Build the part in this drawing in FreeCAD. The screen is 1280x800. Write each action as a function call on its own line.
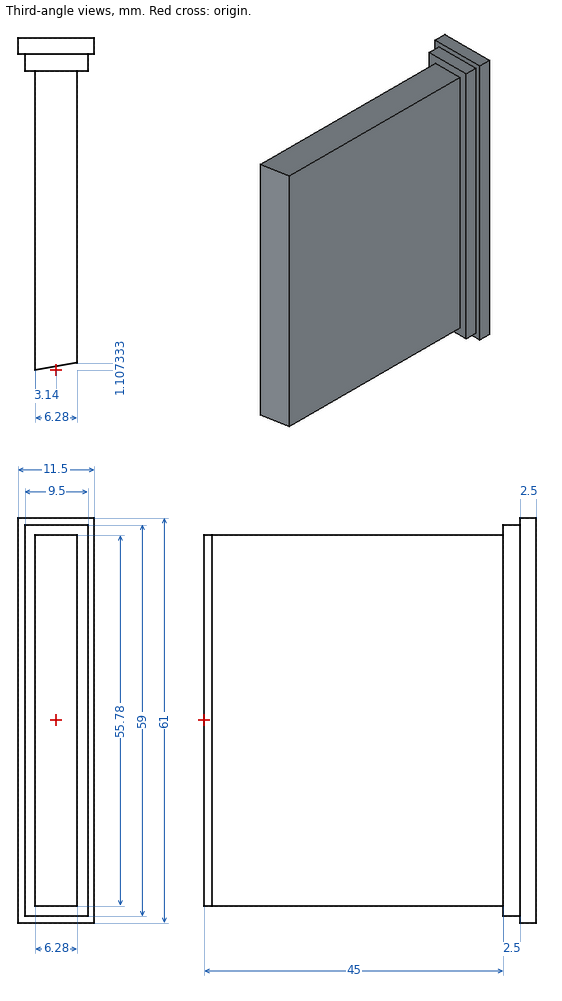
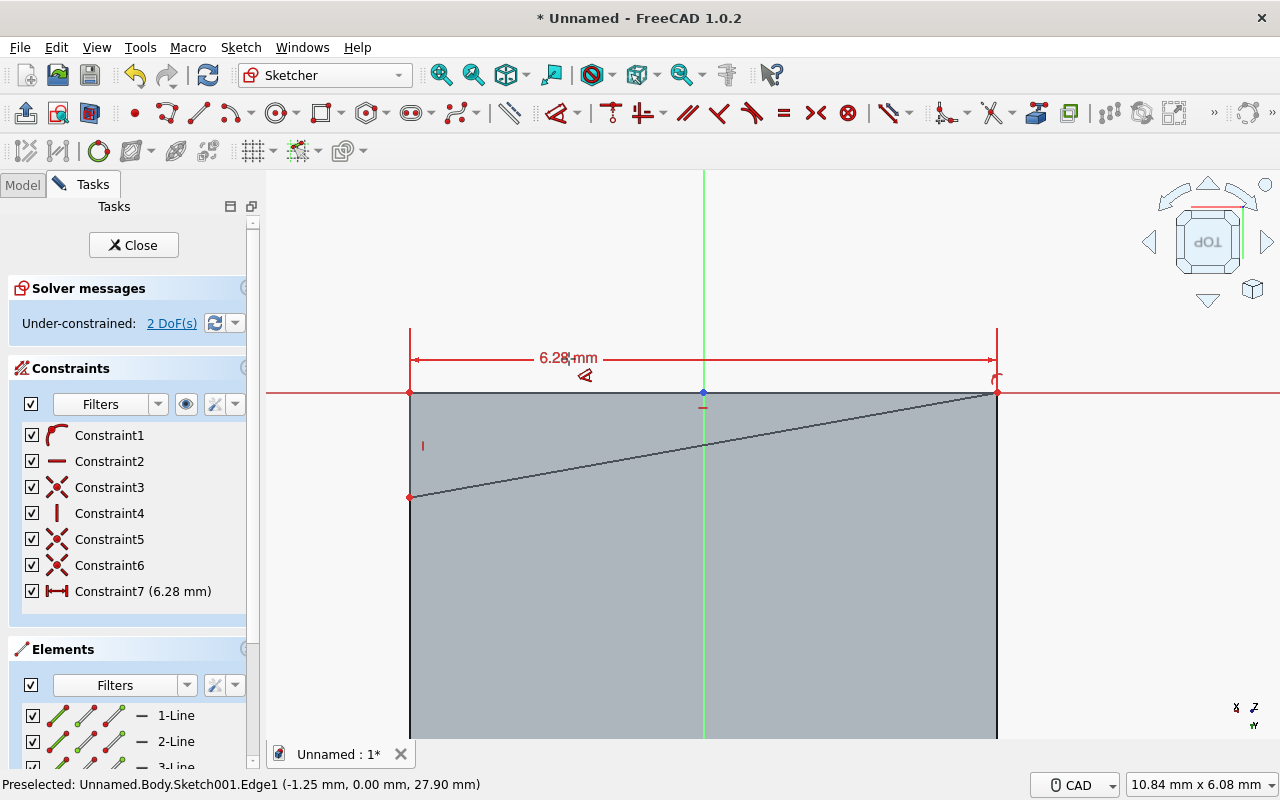
click(997, 393)
click(850, 359)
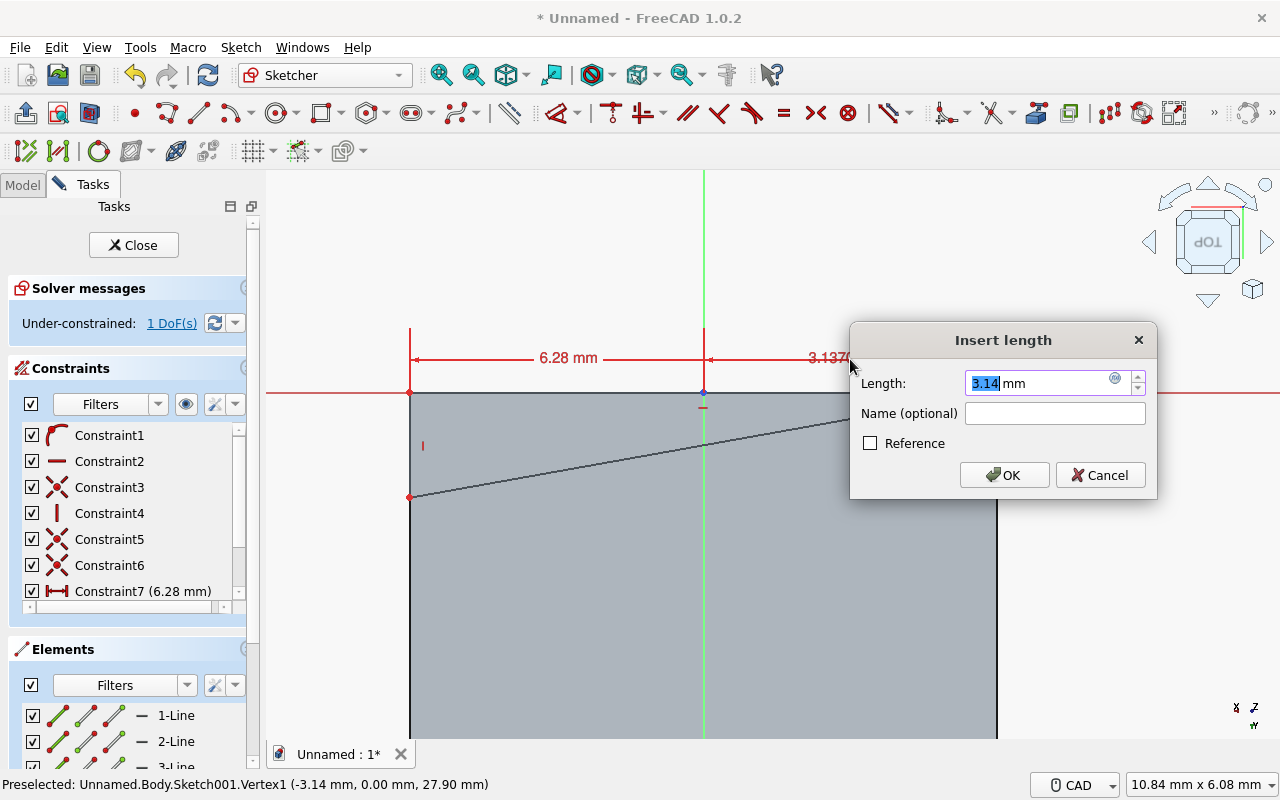
text(3.14)
key(Return)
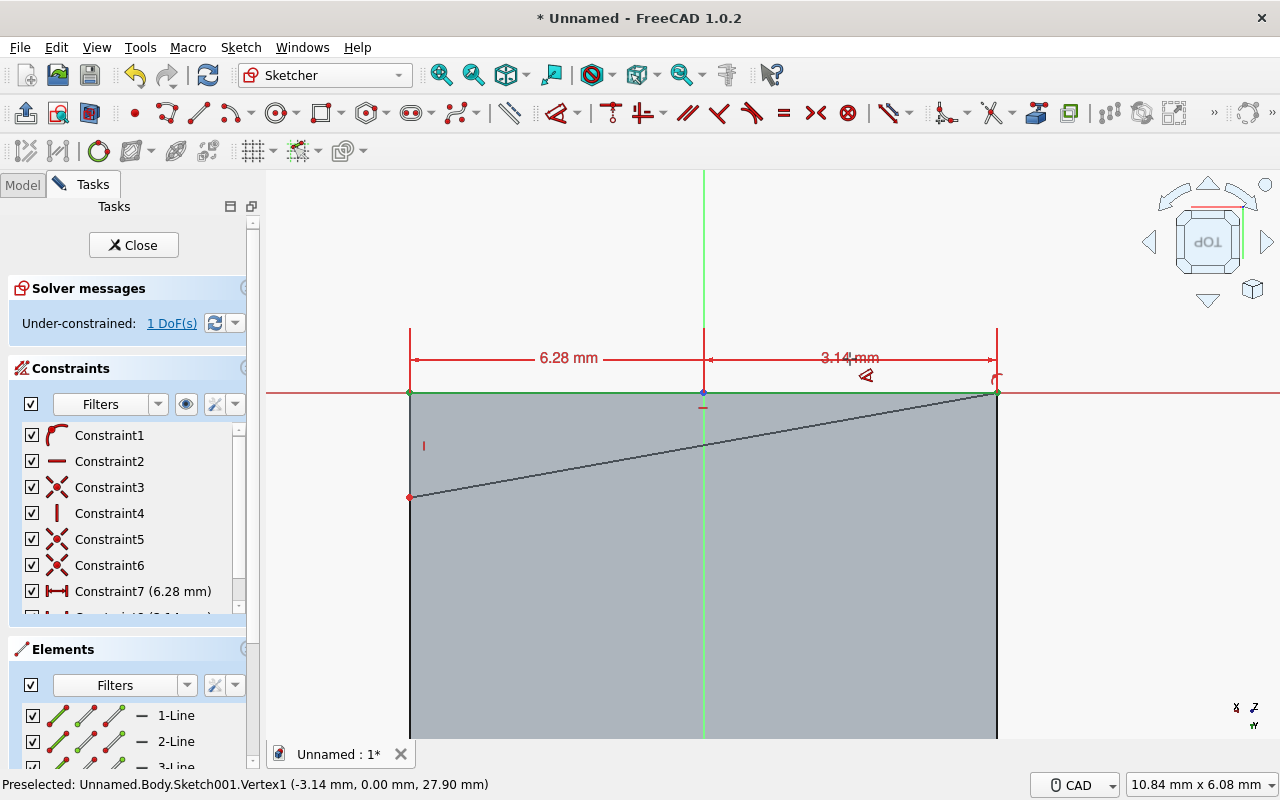
click(410, 424)
click(376, 445)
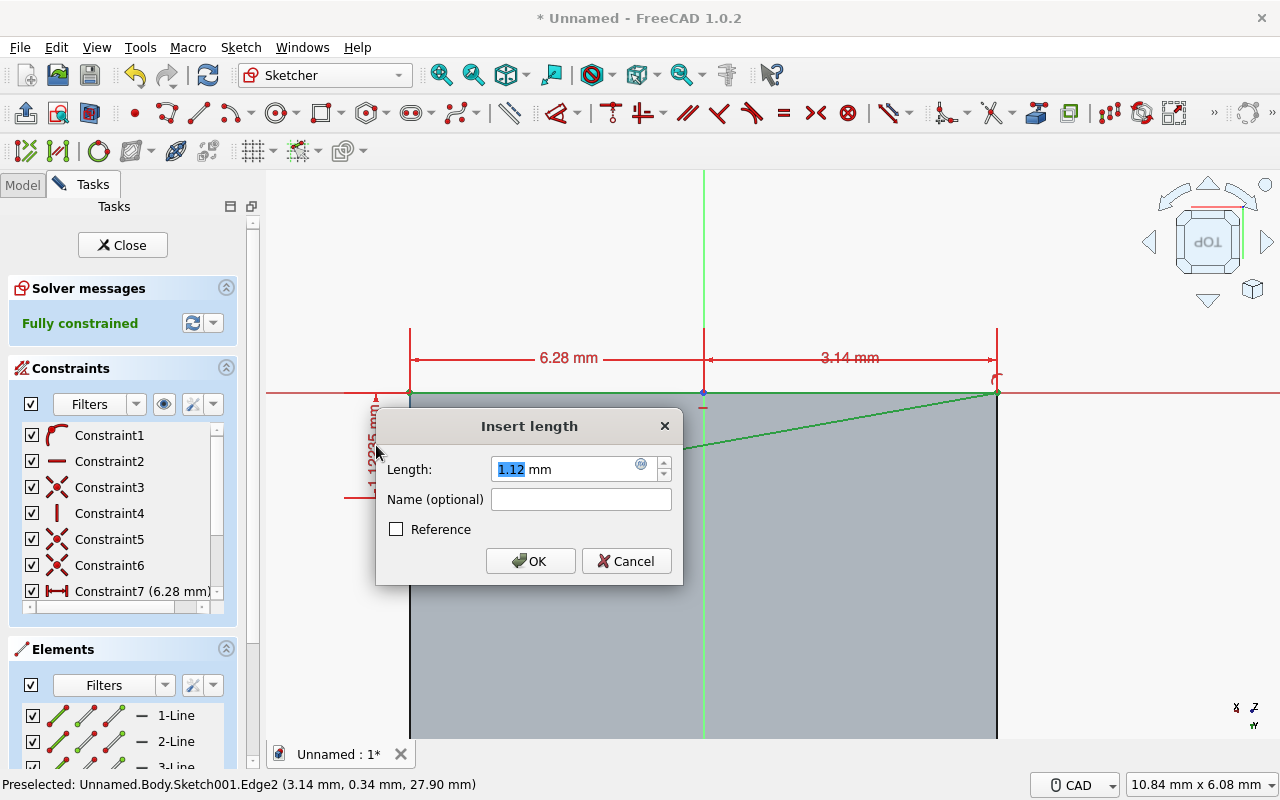
text(1.107333)
key(Return)
key(Escape)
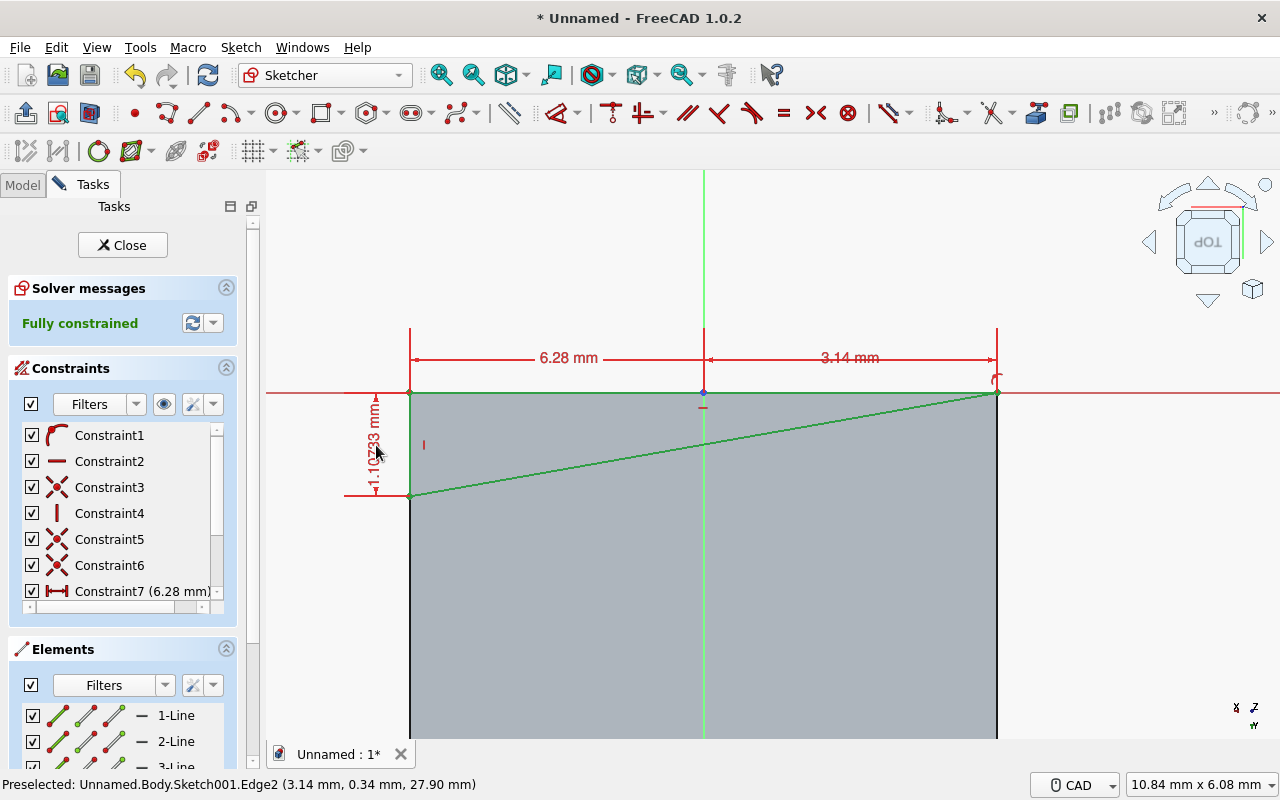
click(123, 245)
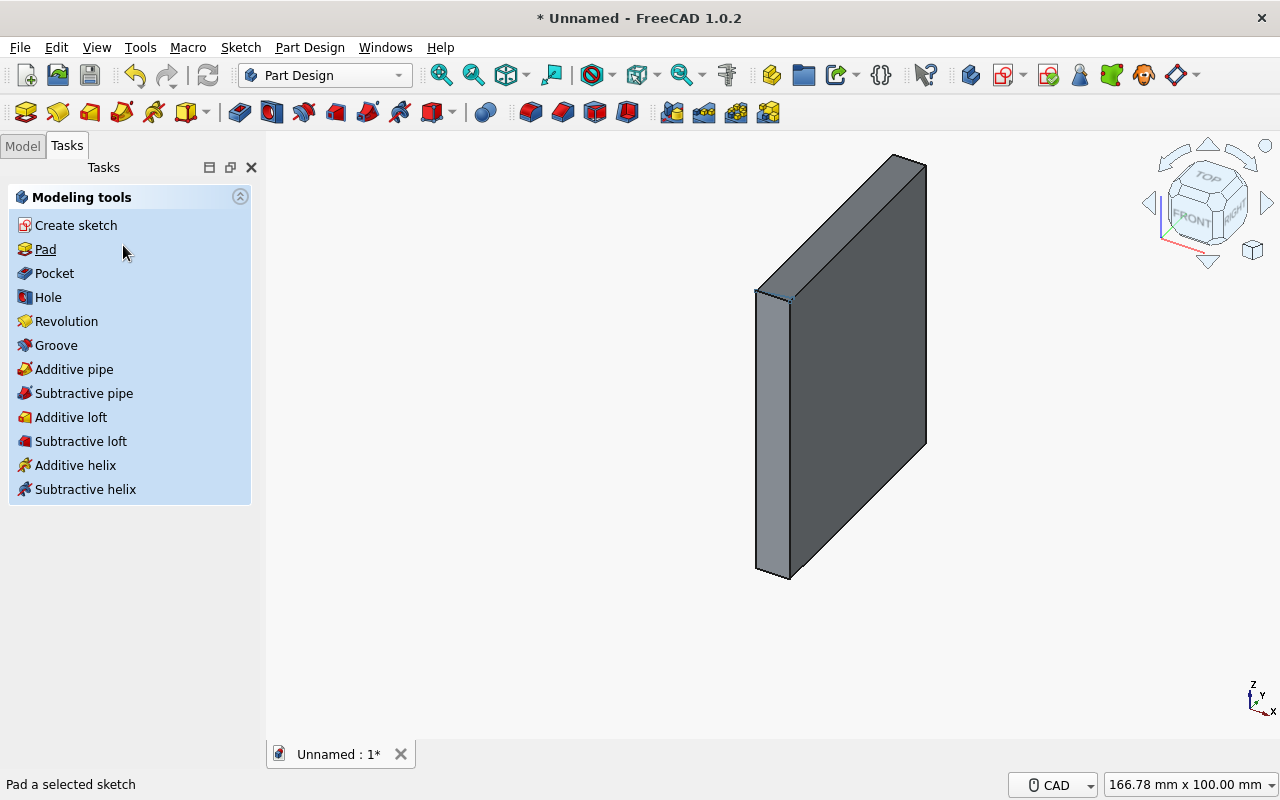
click(240, 112)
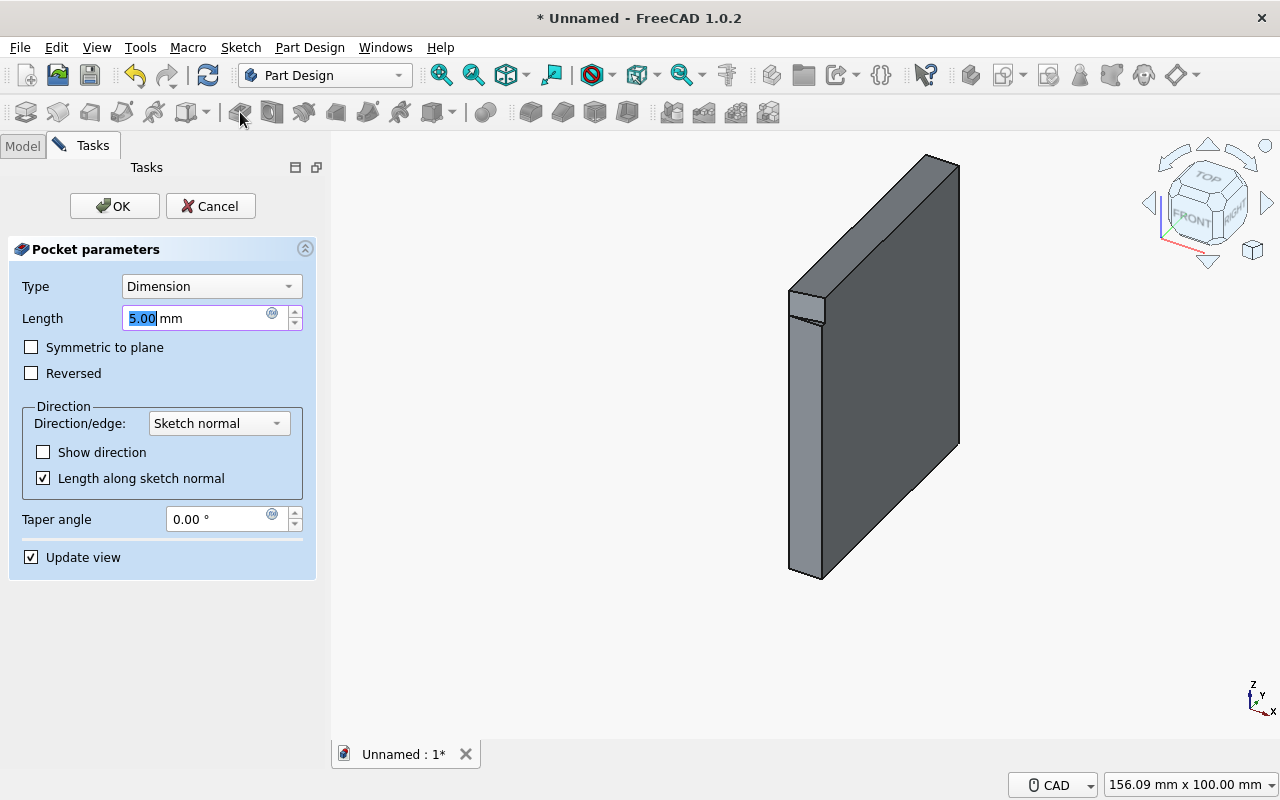
click(212, 286)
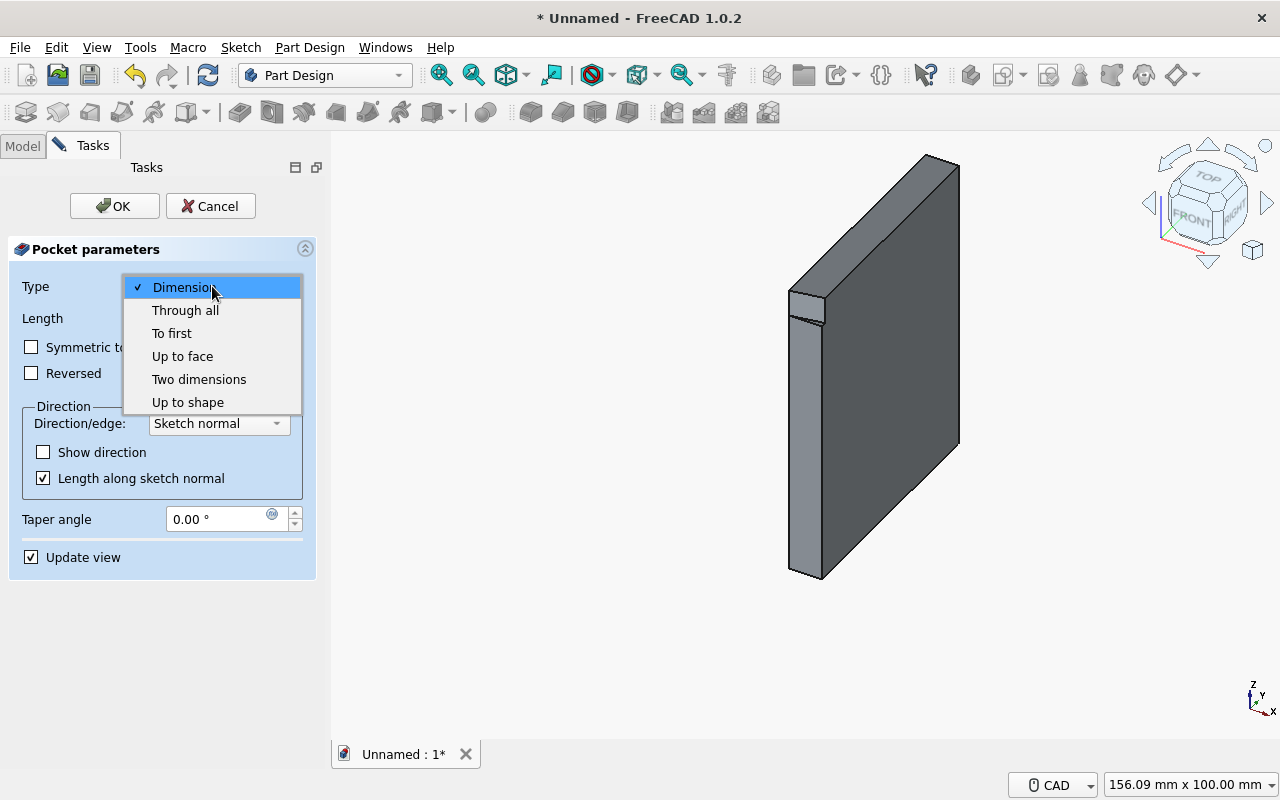
click(212, 310)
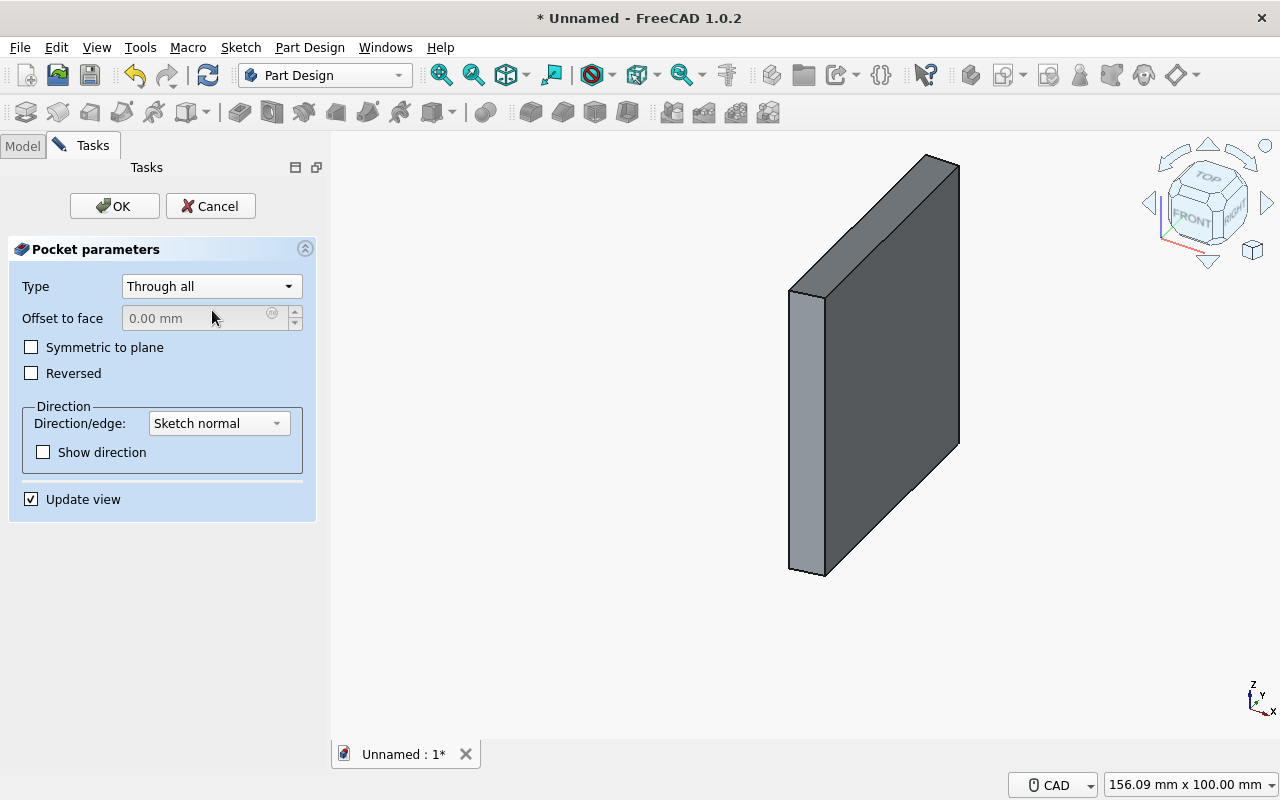
click(115, 206)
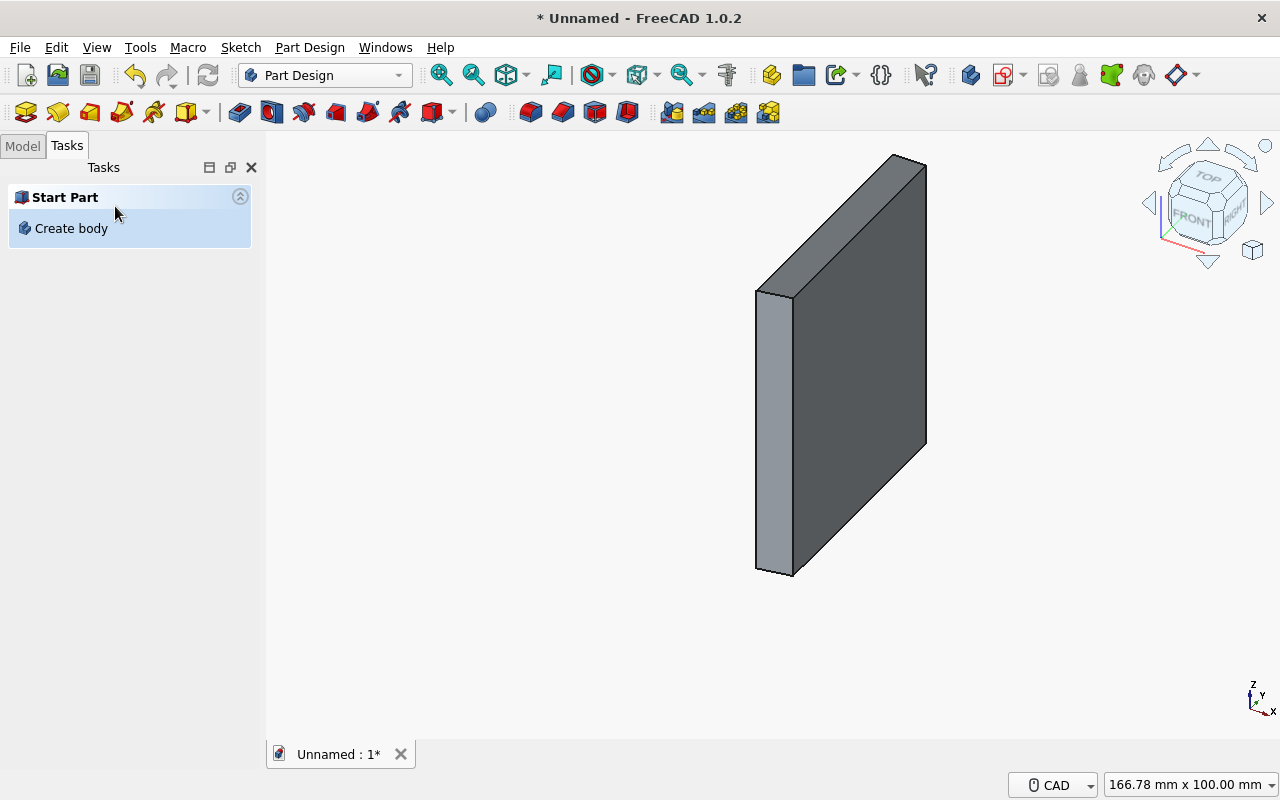
key(4)